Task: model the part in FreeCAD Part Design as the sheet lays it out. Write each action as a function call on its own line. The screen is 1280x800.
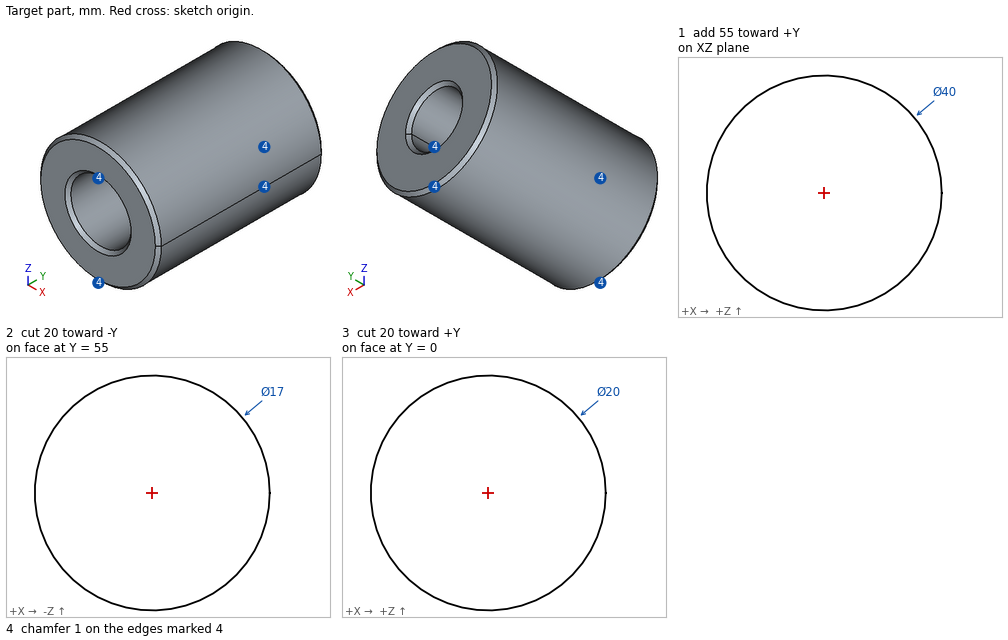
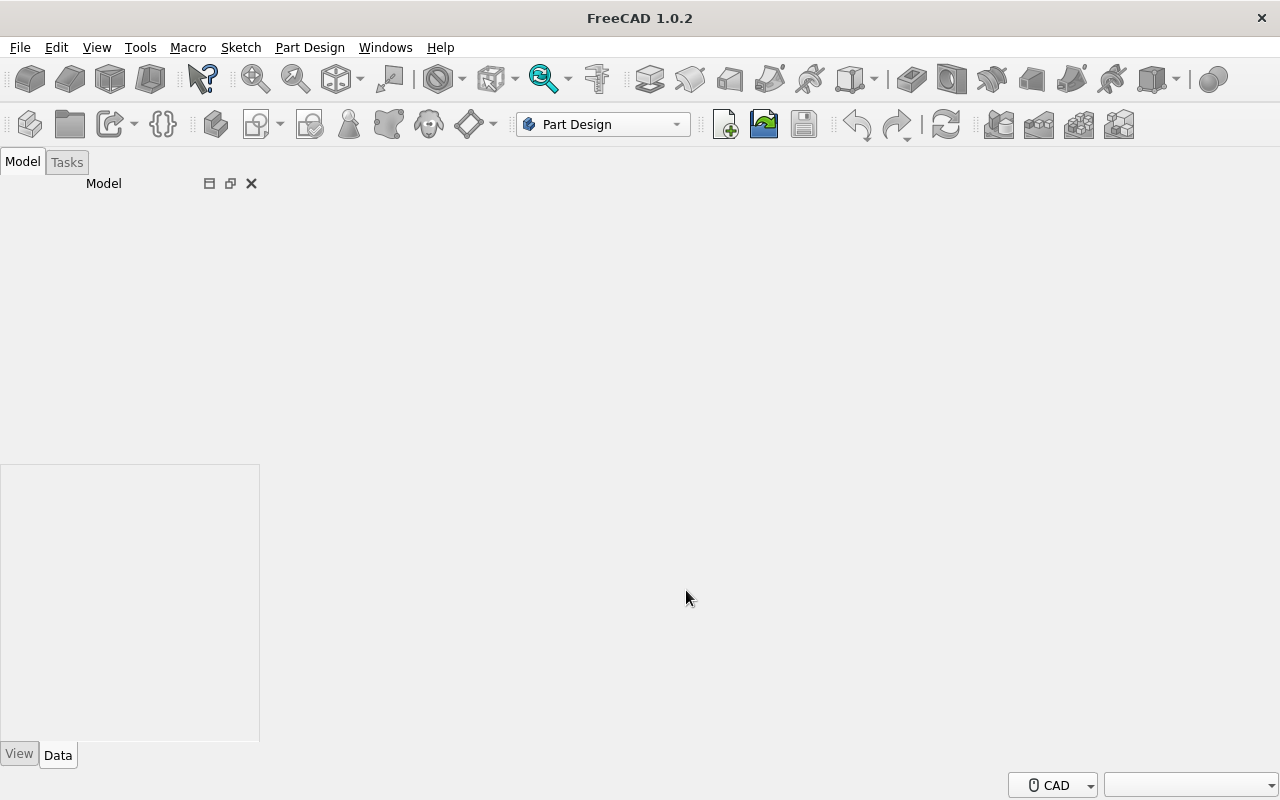
click(724, 124)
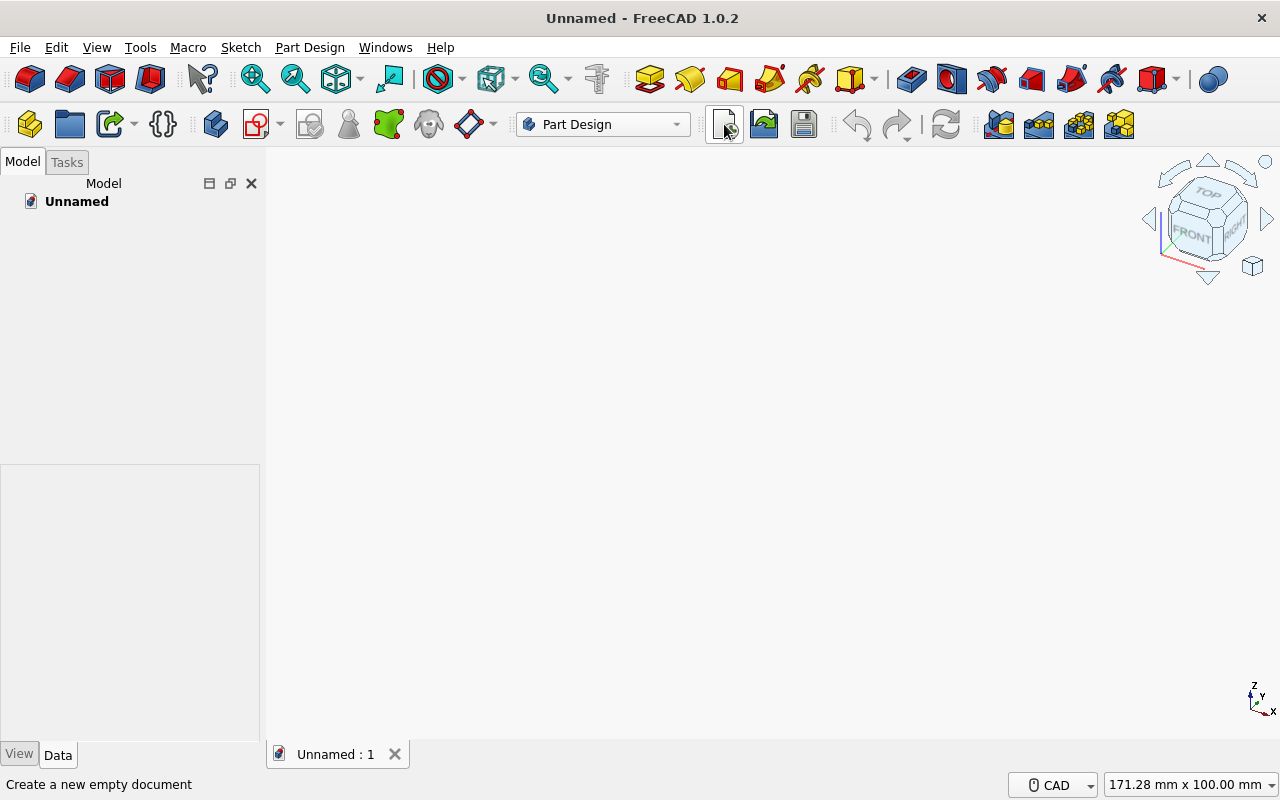
click(256, 124)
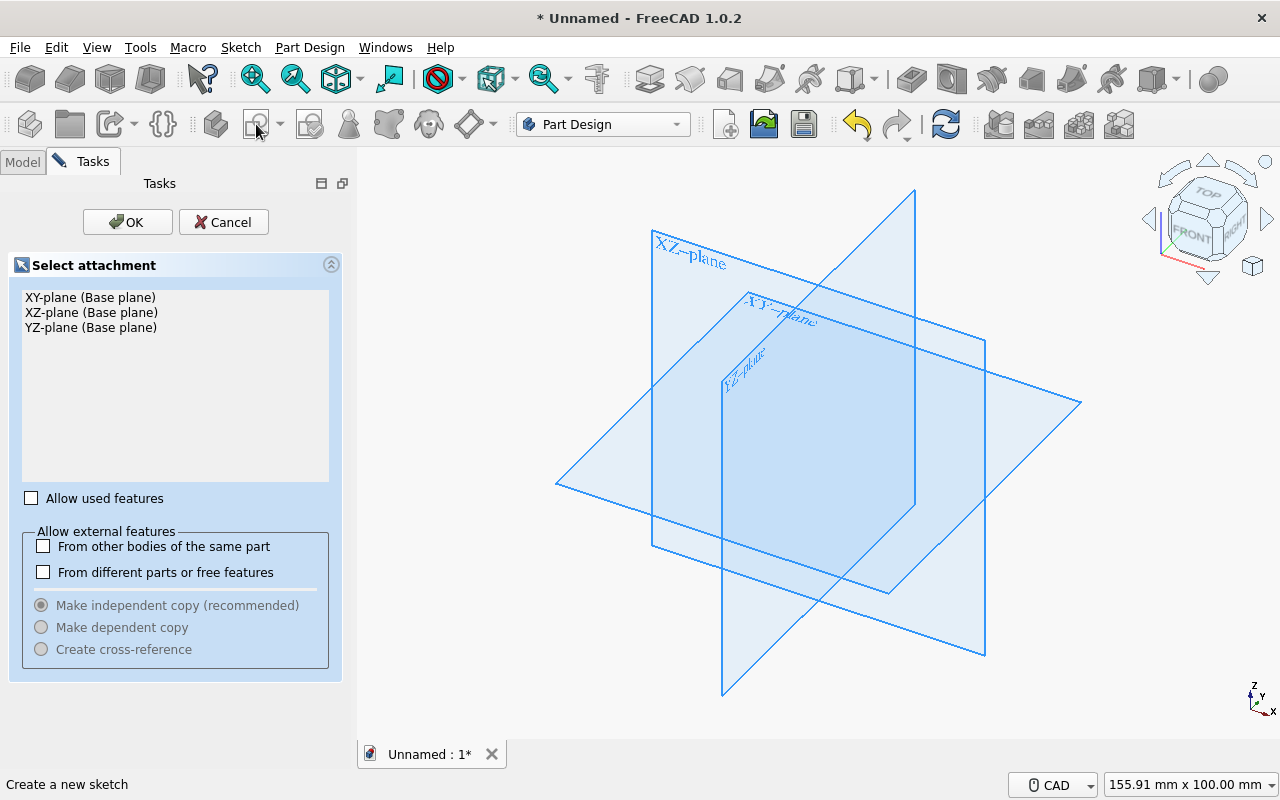
click(82, 312)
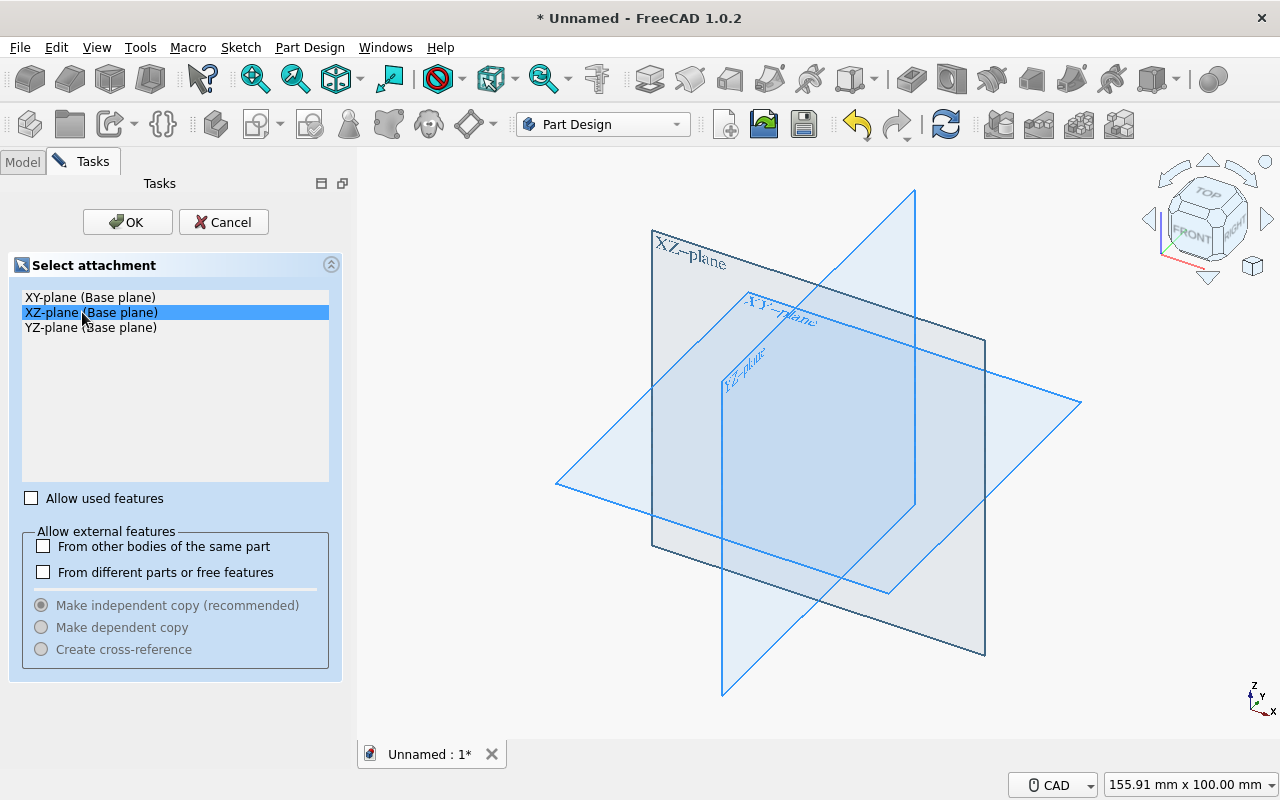
click(128, 222)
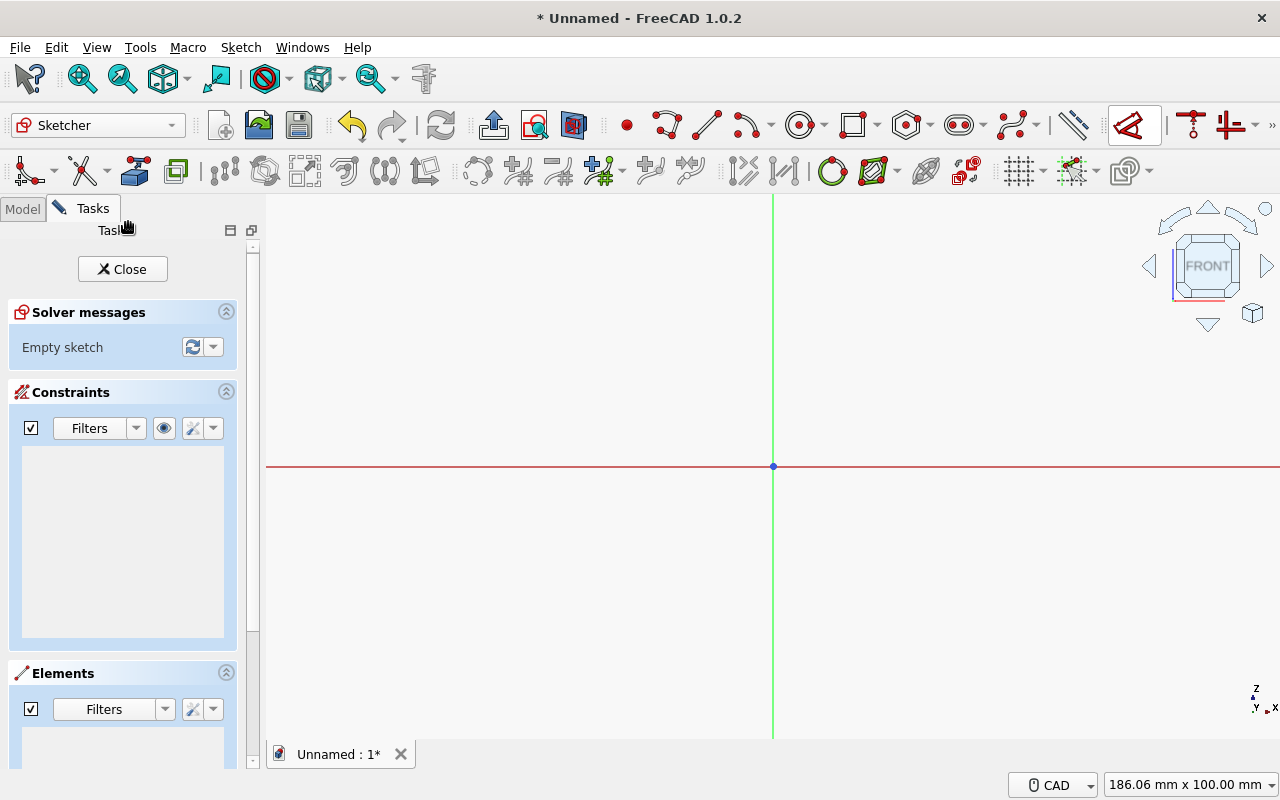
scroll(912, 467, up, 2)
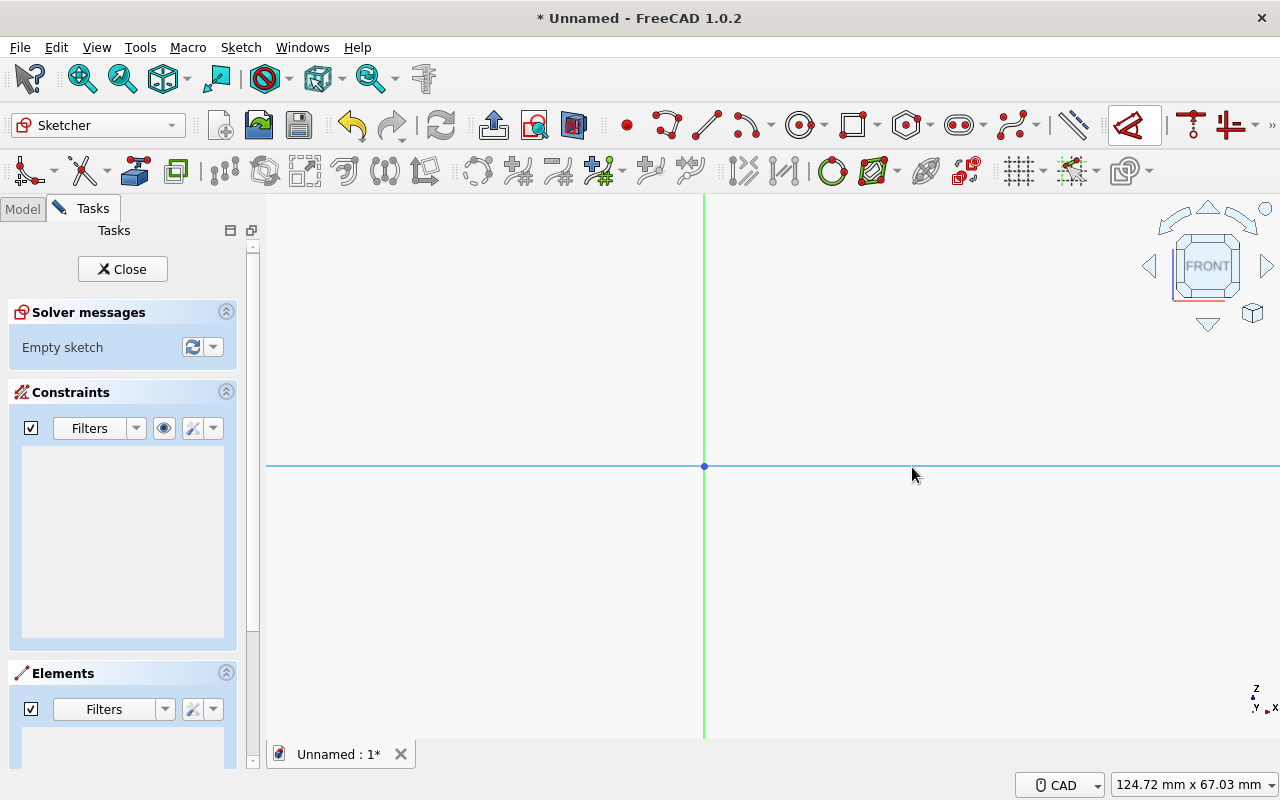
click(800, 126)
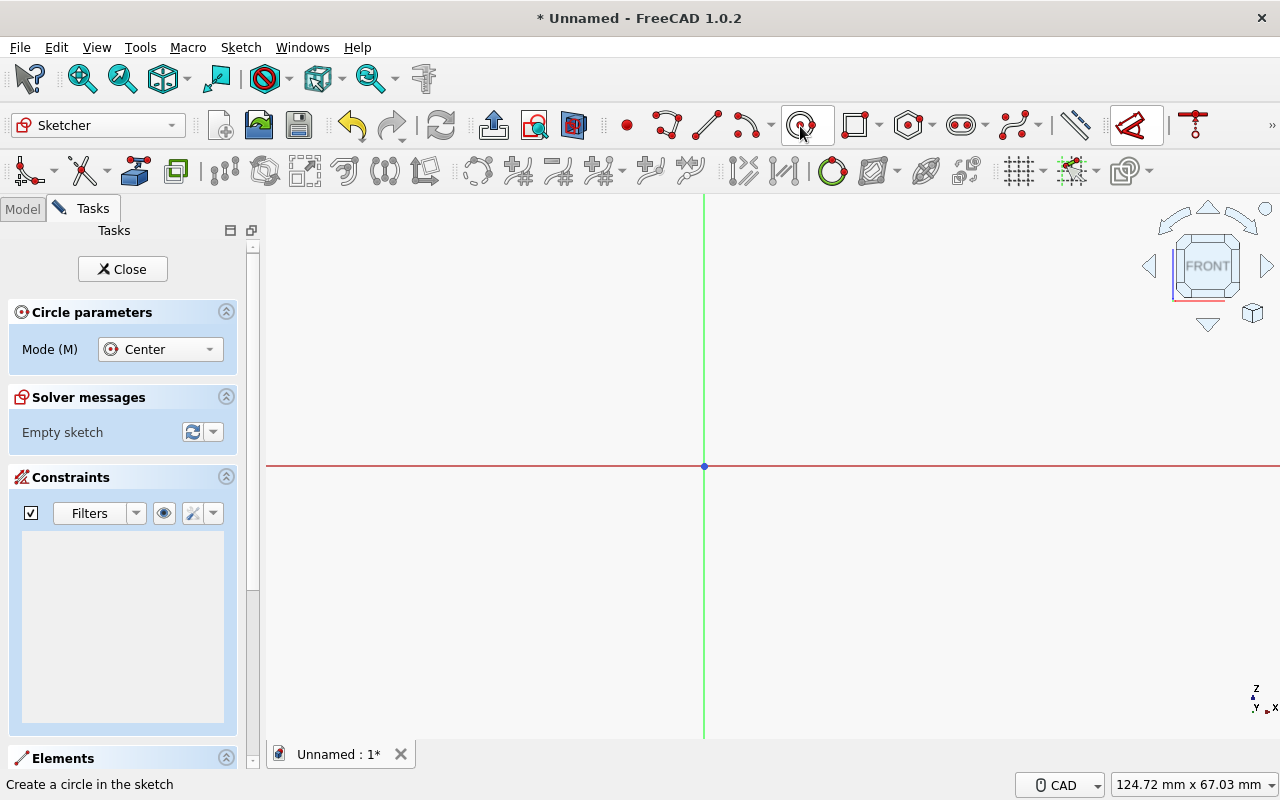
click(704, 466)
move(819, 351)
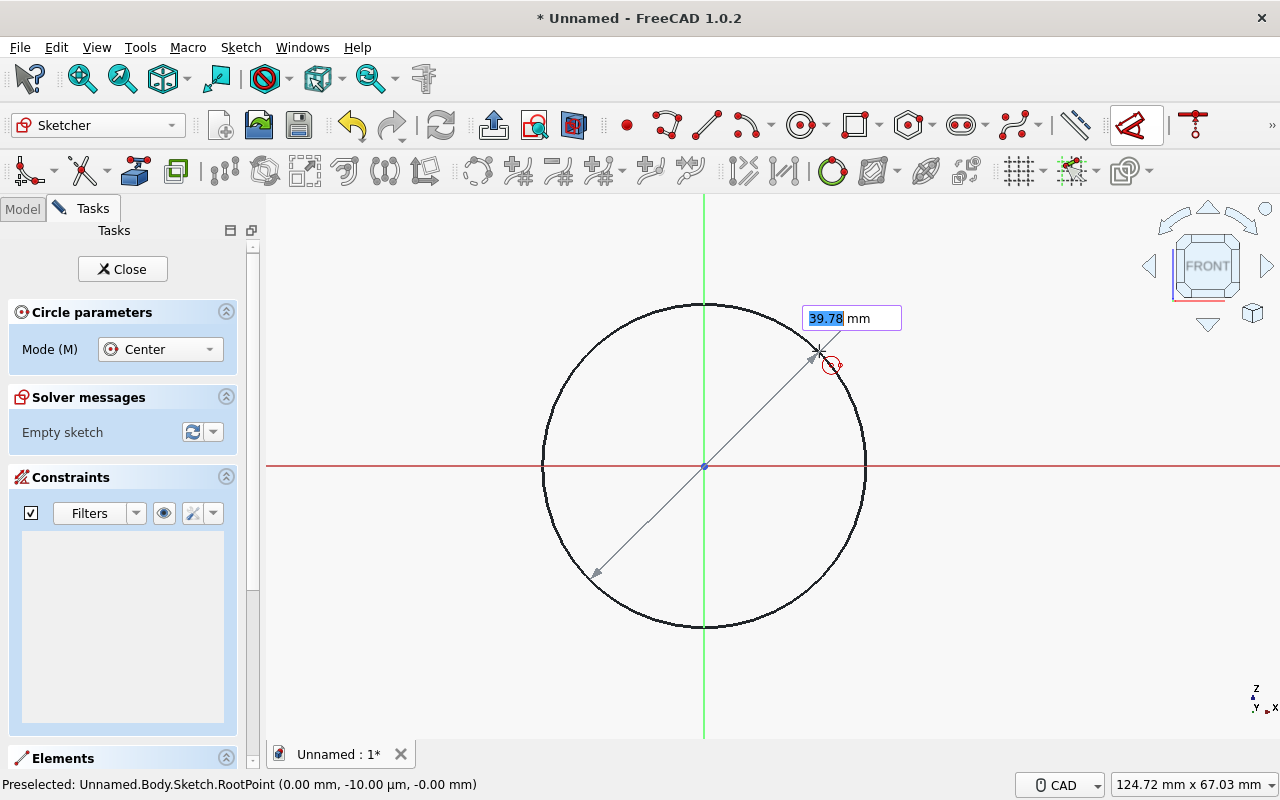
text(40)
key(Return)
key(Escape)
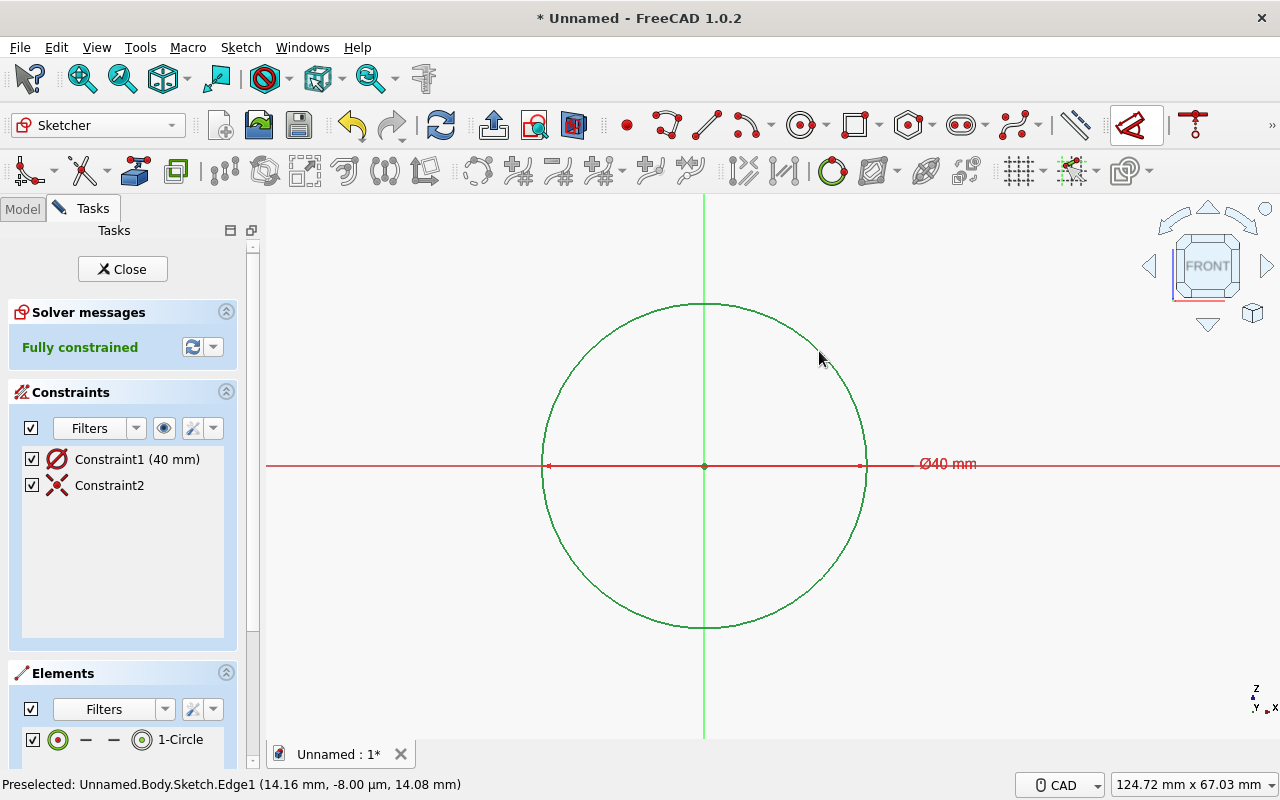
click(123, 269)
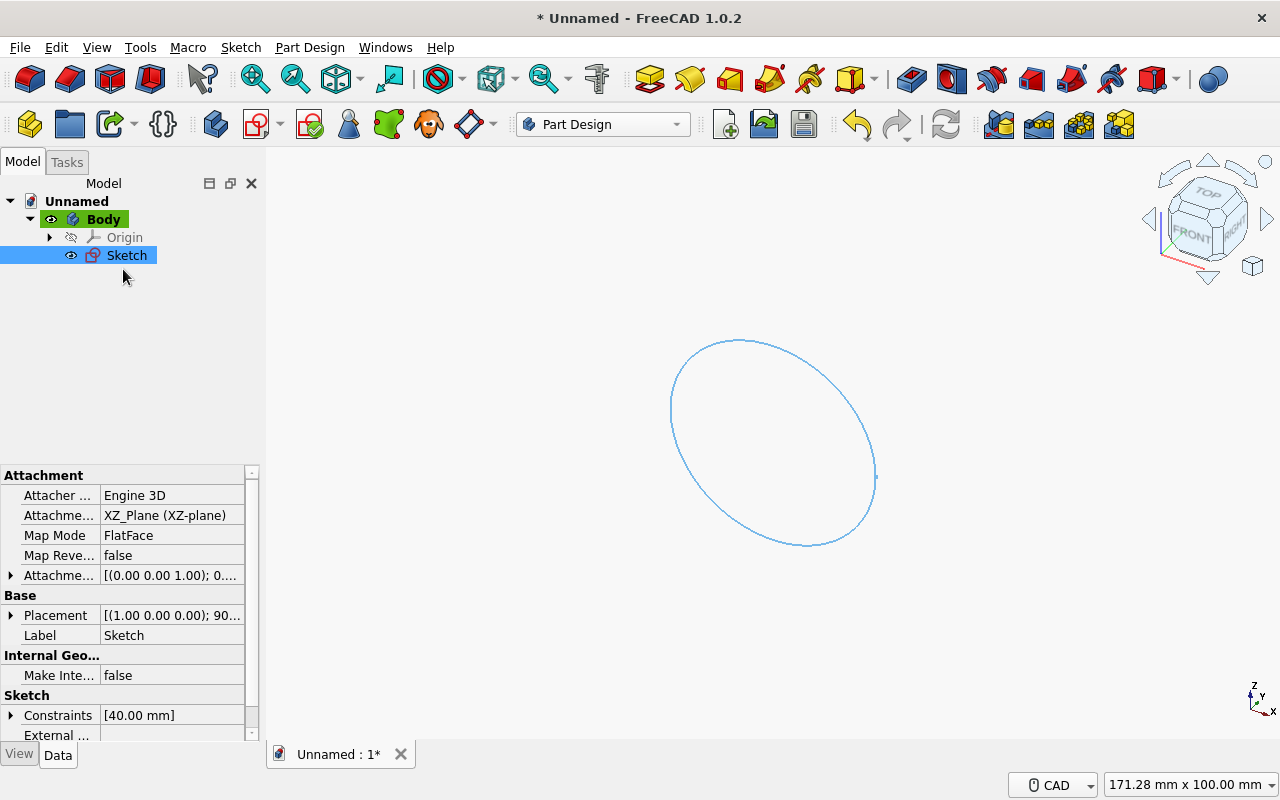
click(650, 80)